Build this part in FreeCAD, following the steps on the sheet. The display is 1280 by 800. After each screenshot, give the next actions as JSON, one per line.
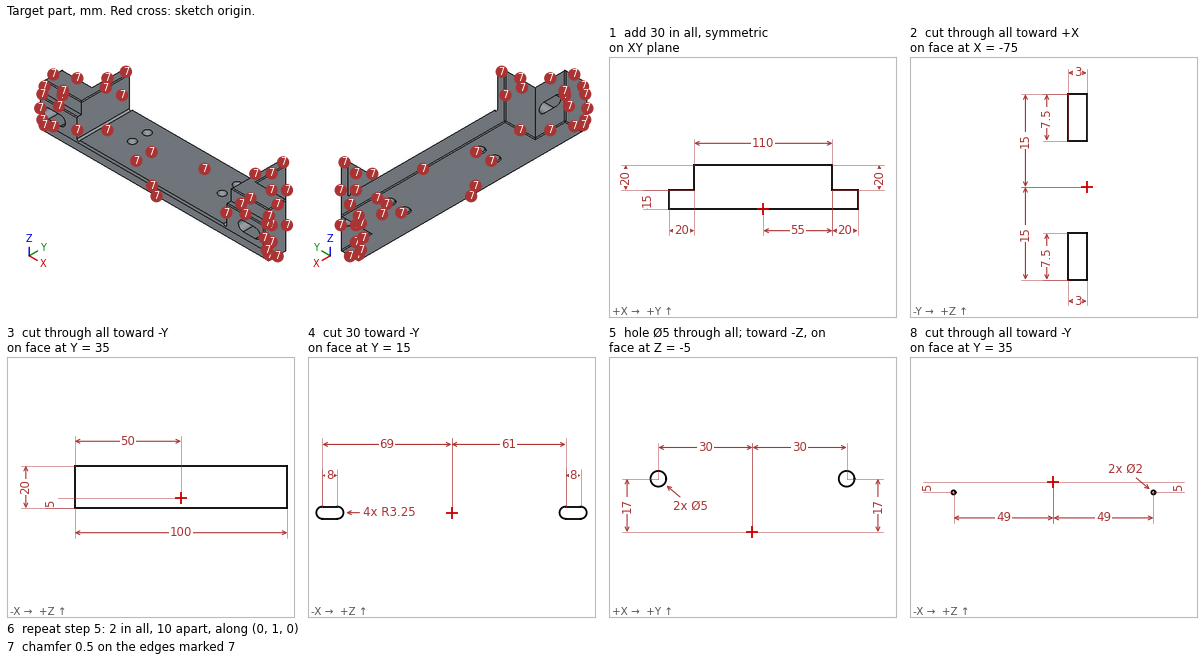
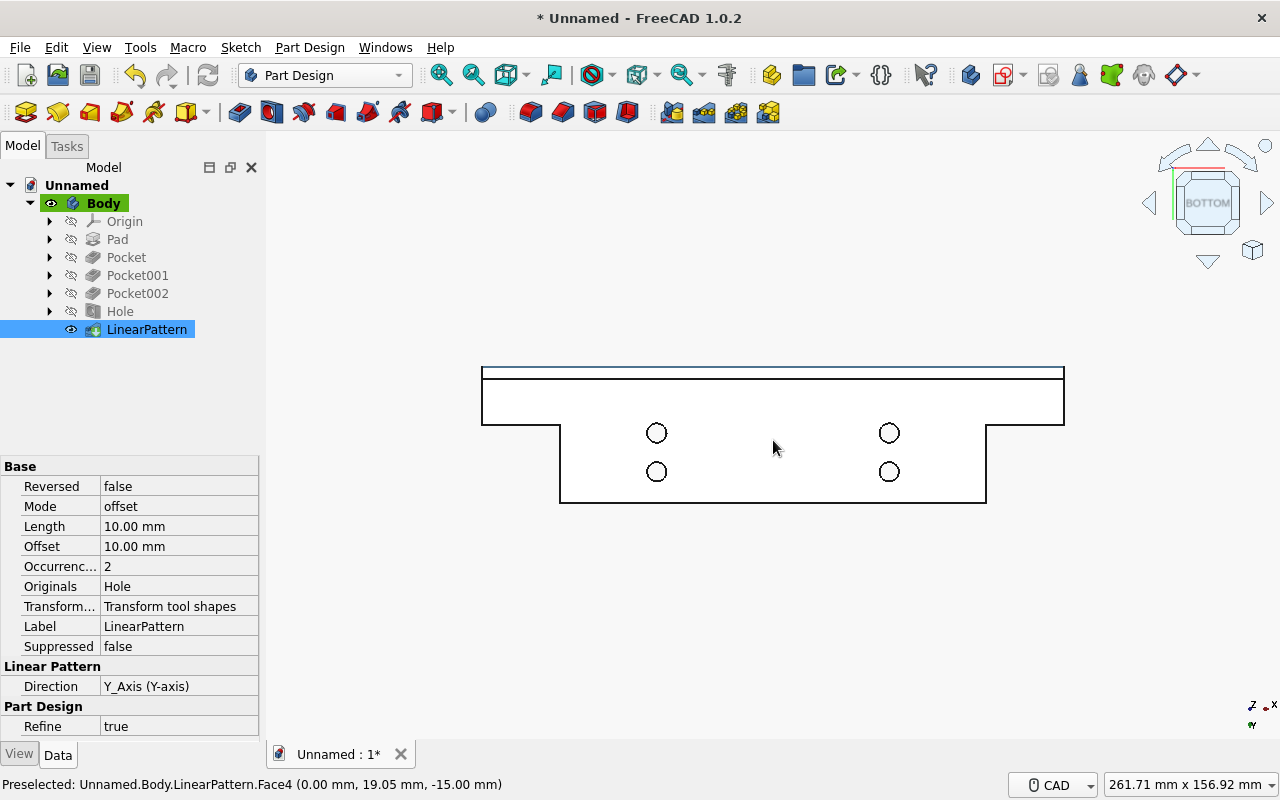
{"action": "key", "text": "4"}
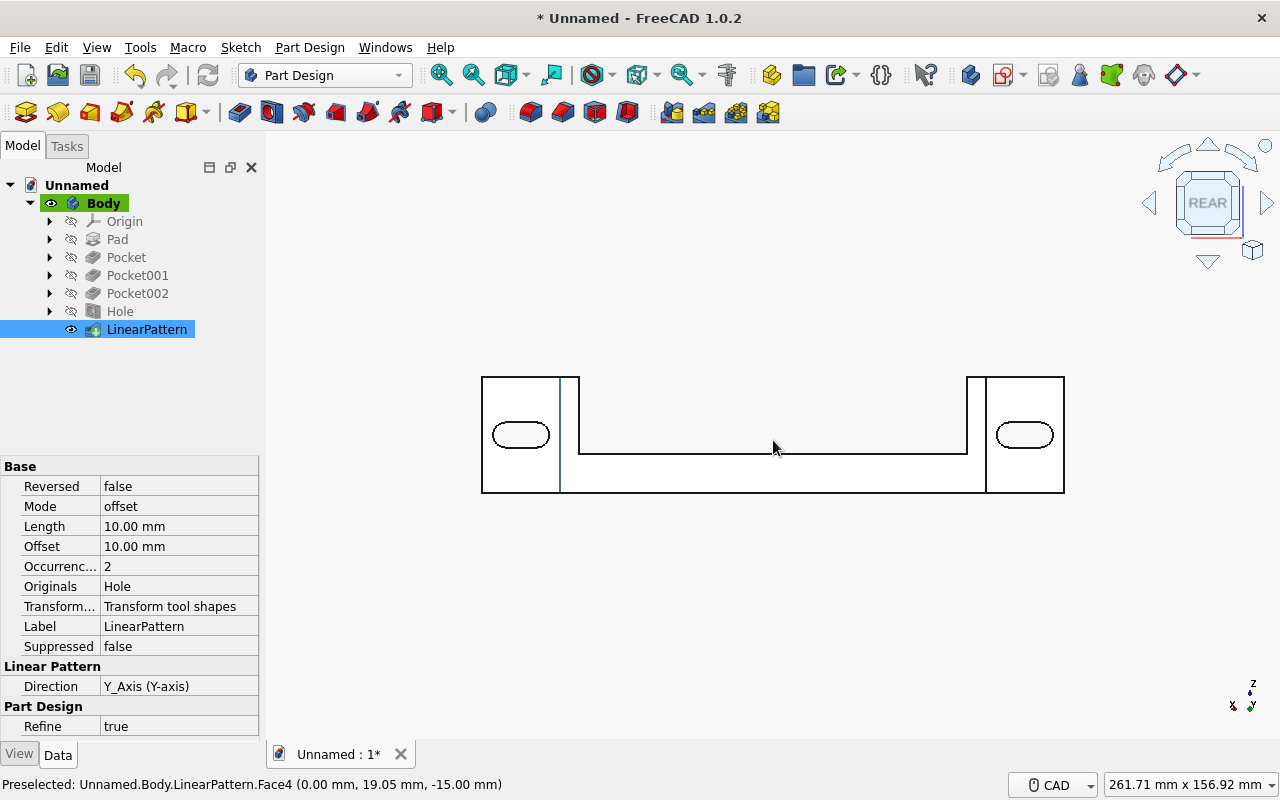
{"action": "left_click", "coordinate": [986, 434], "text": "ctrl"}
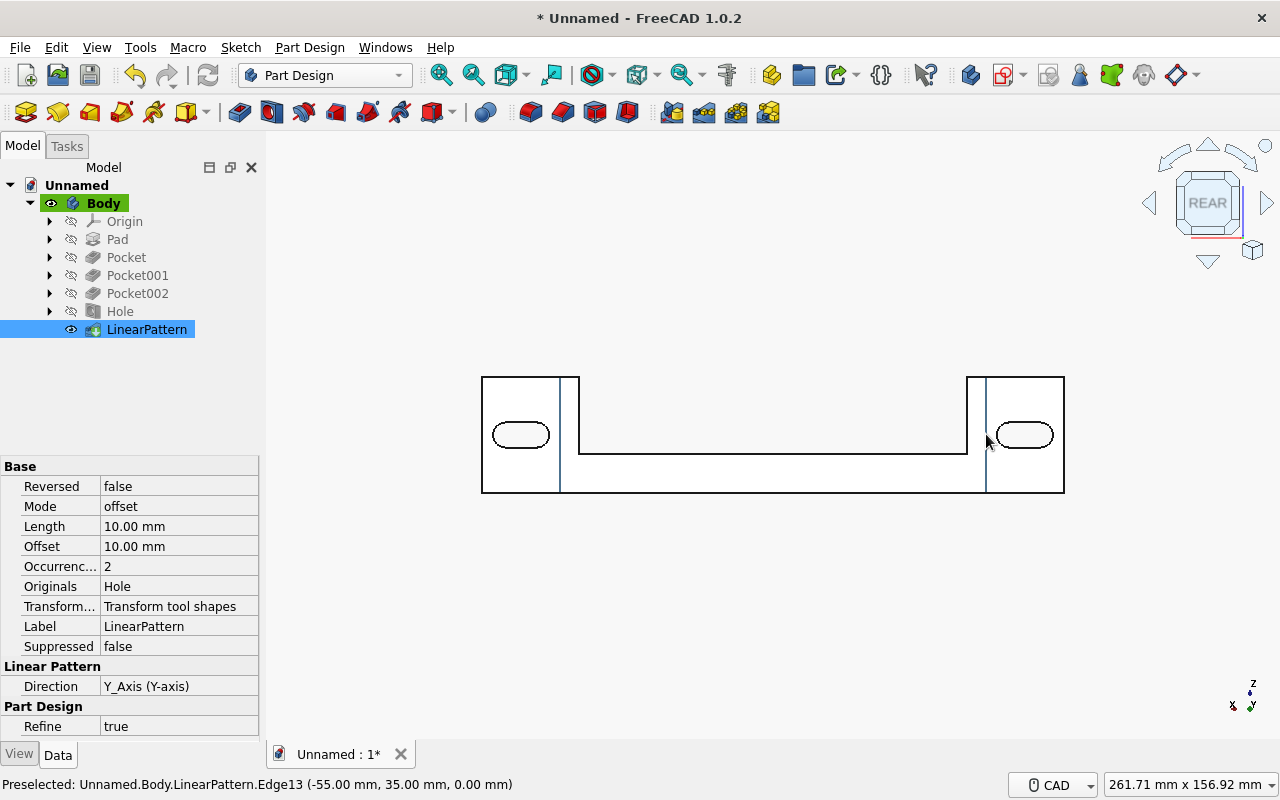
{"action": "key", "text": "6"}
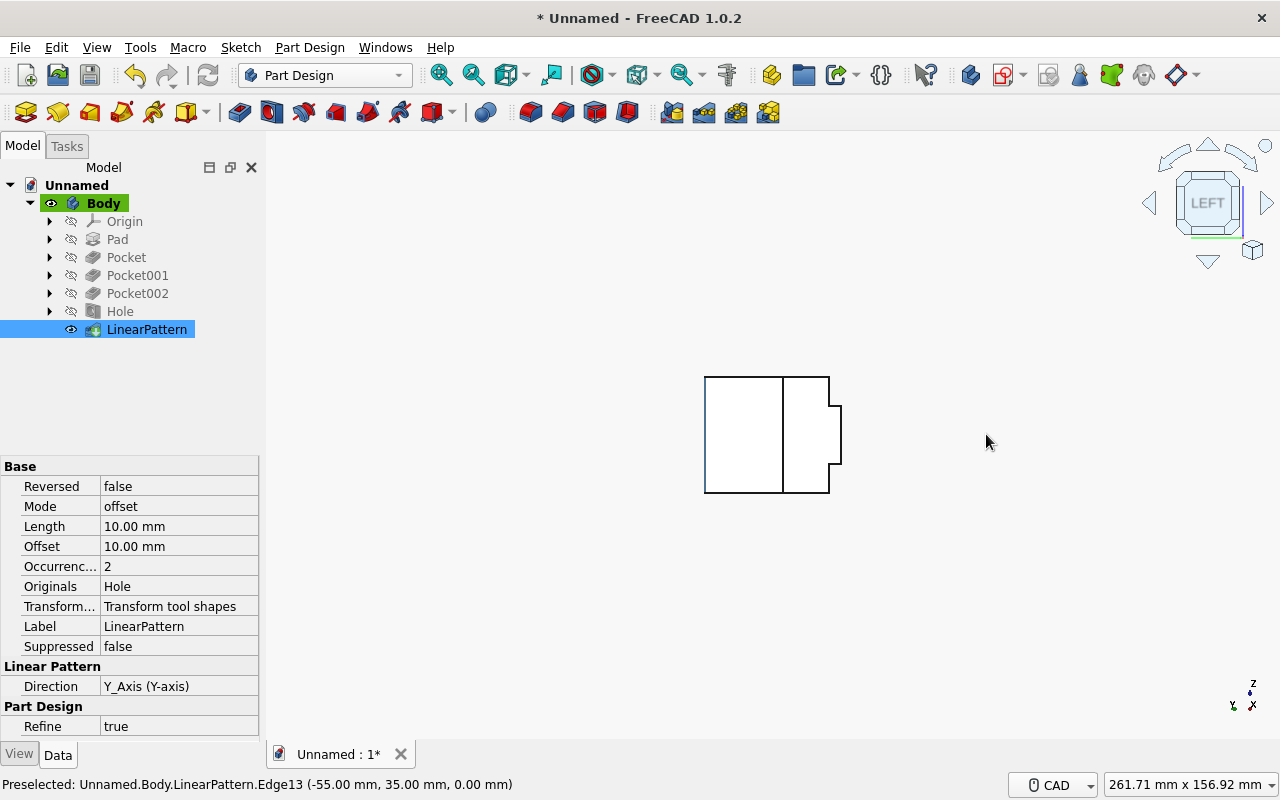
{"action": "key", "text": "v f"}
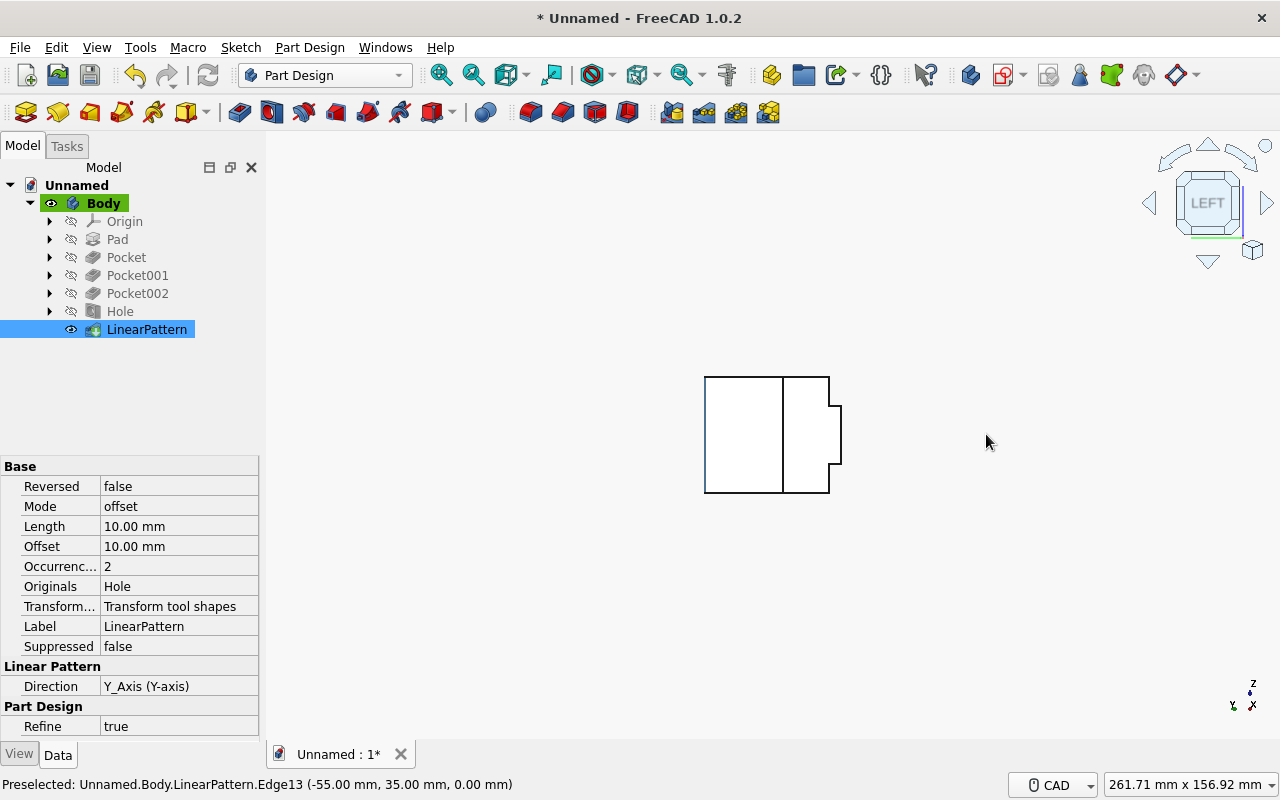
{"action": "left_click", "coordinate": [812, 434], "text": "ctrl"}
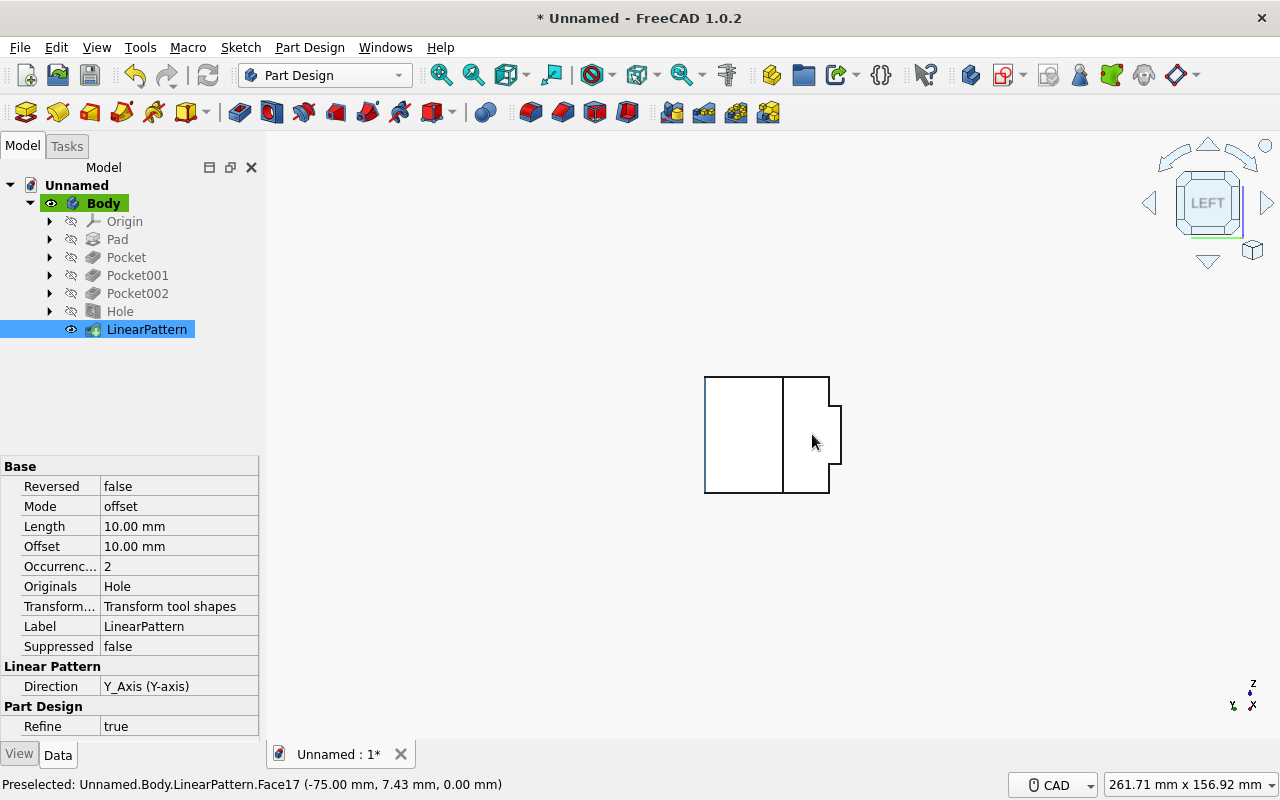
{"action": "left_click", "coordinate": [564, 112]}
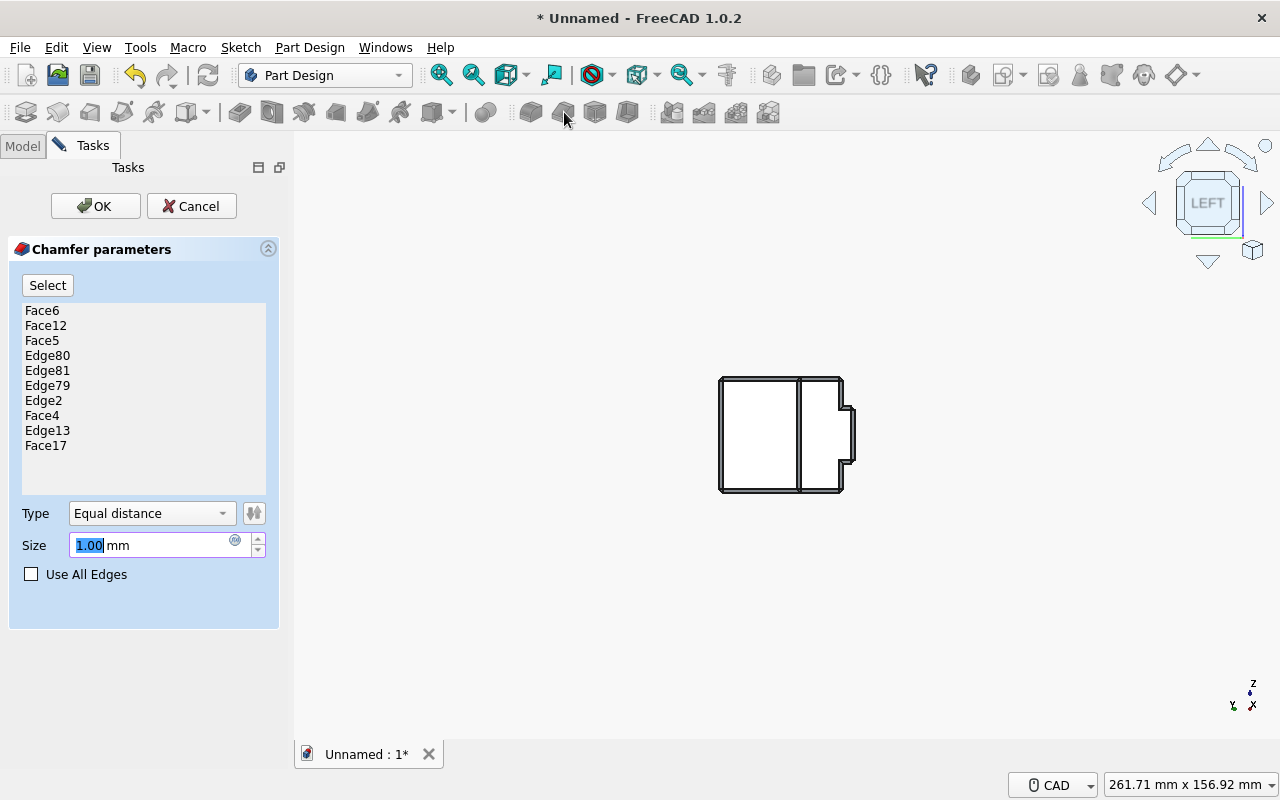
{"action": "type", "text": "0.5"}
{"action": "key", "text": "Tab"}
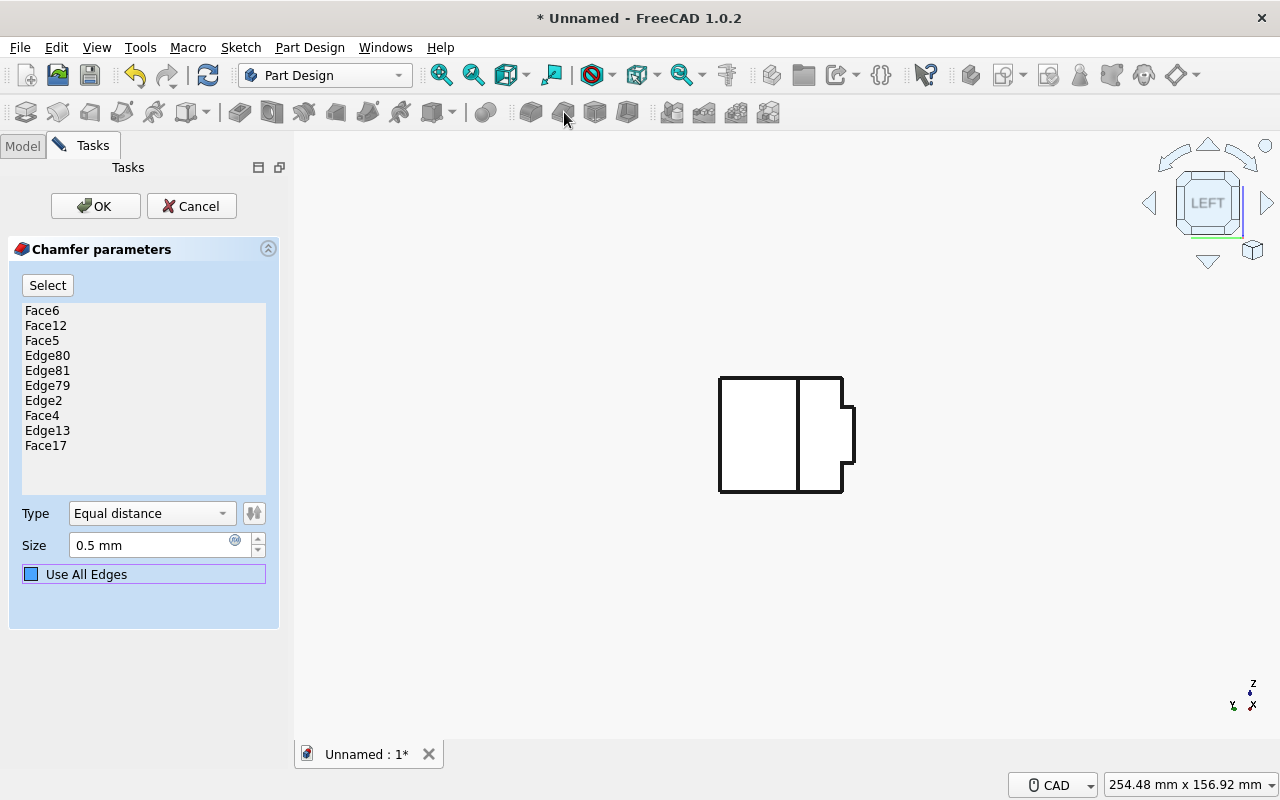
{"action": "left_click", "coordinate": [96, 206]}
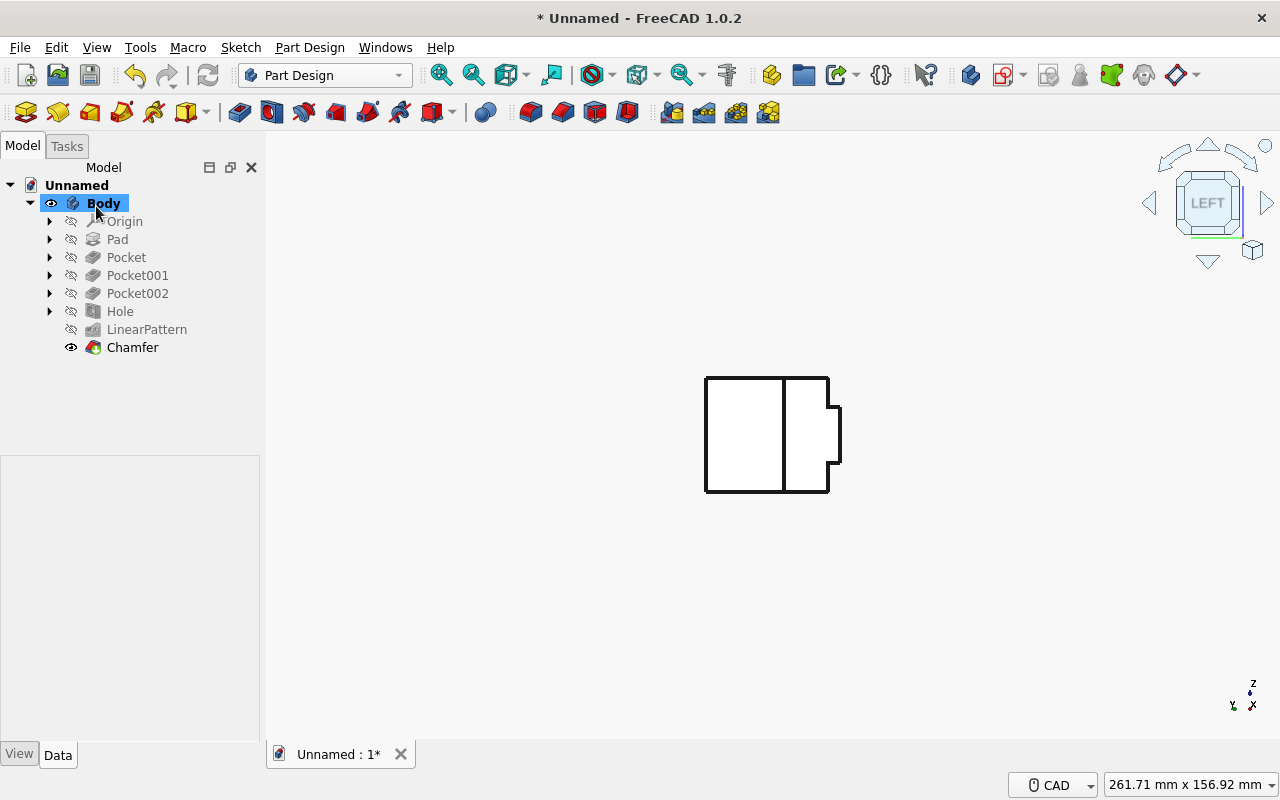
{"action": "left_click", "coordinate": [442, 76]}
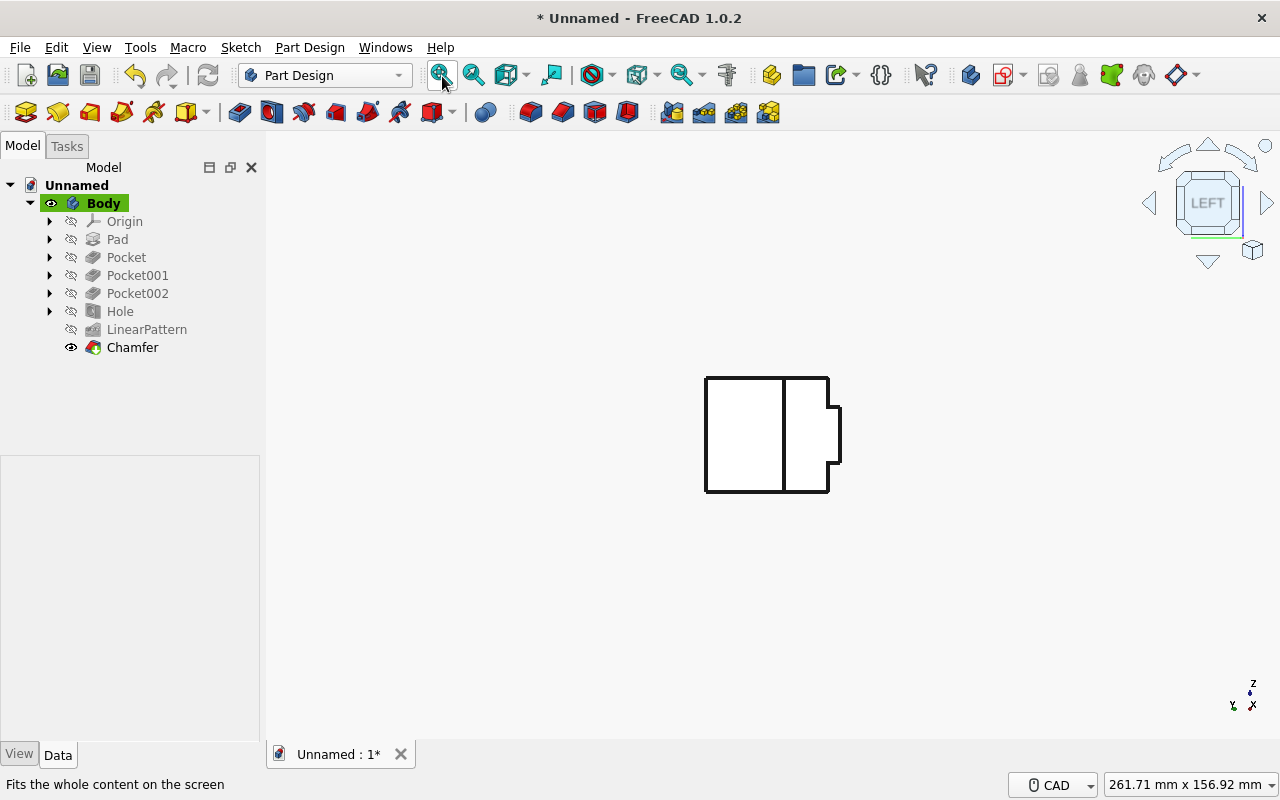
{"action": "key", "text": "4"}